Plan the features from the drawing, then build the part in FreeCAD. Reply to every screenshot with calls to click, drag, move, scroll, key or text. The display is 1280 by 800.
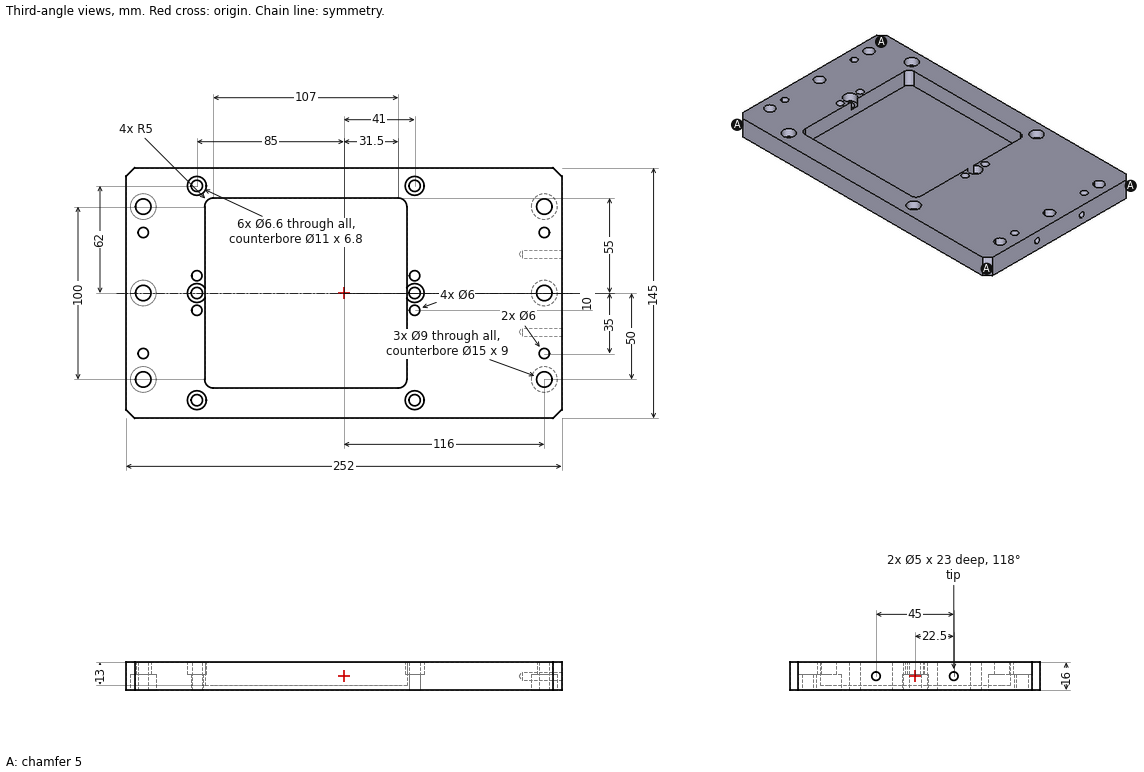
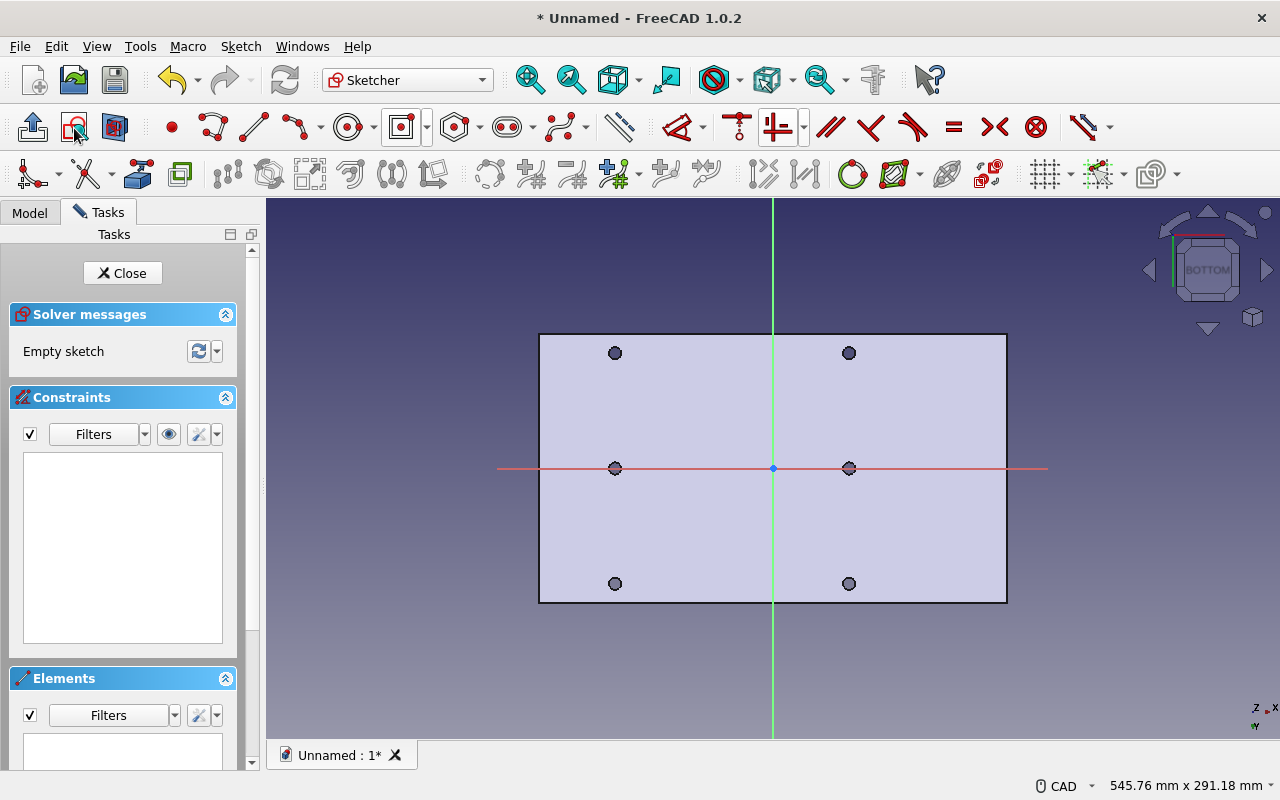
scroll(1104, 468, up, 3)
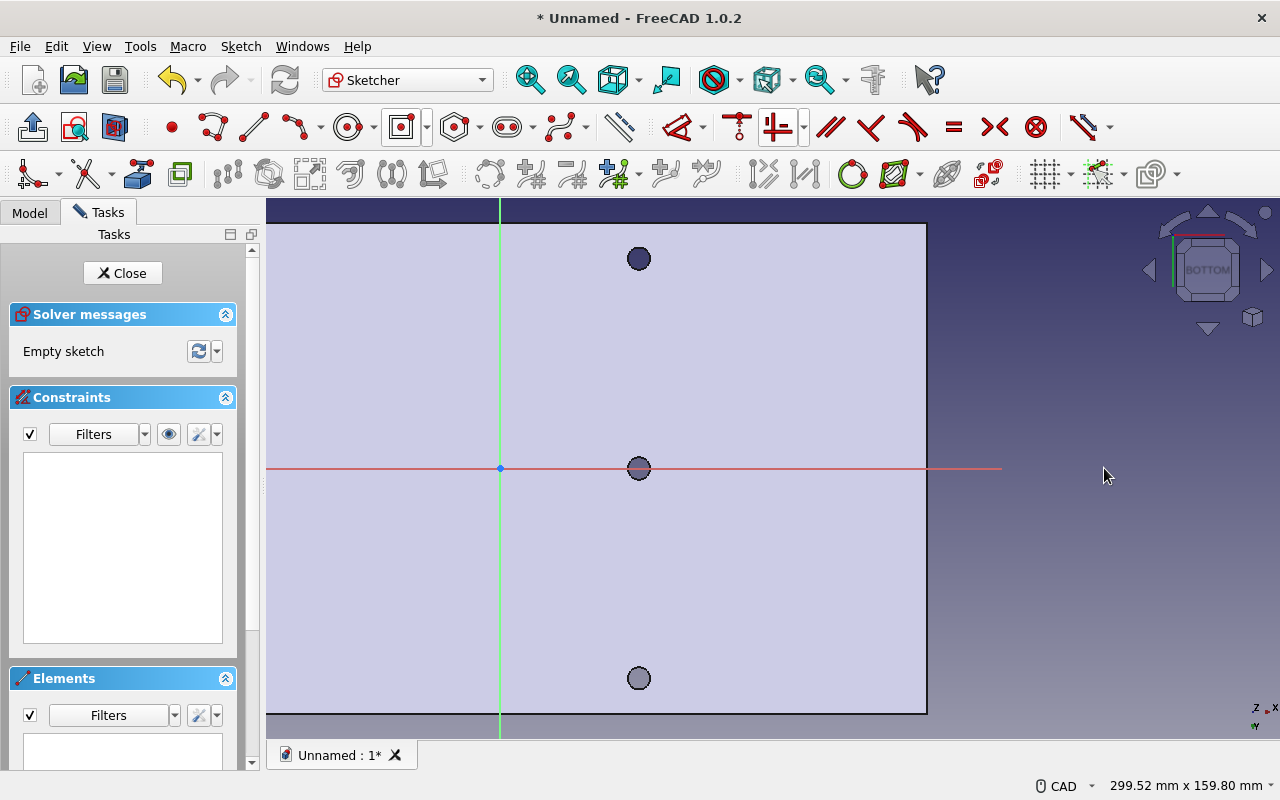
key(g)
key(c)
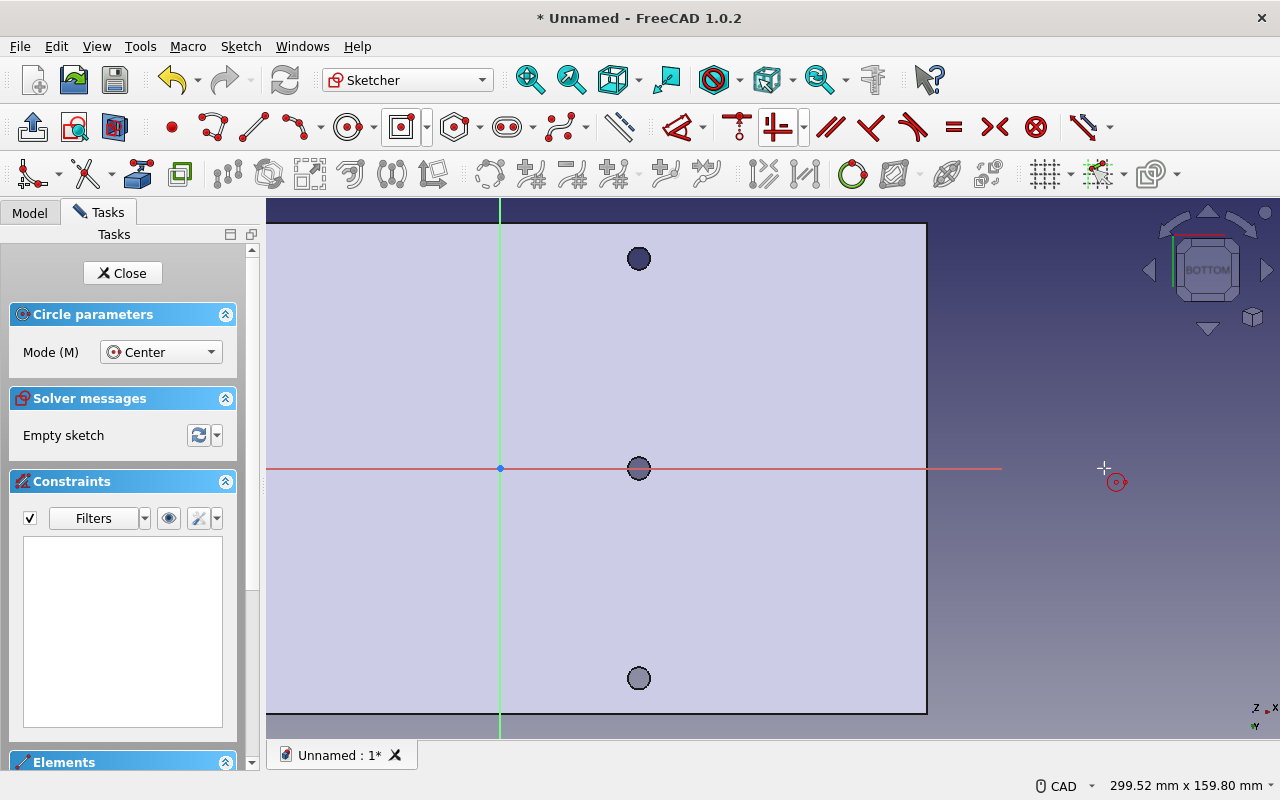
scroll(893, 299, up, 2)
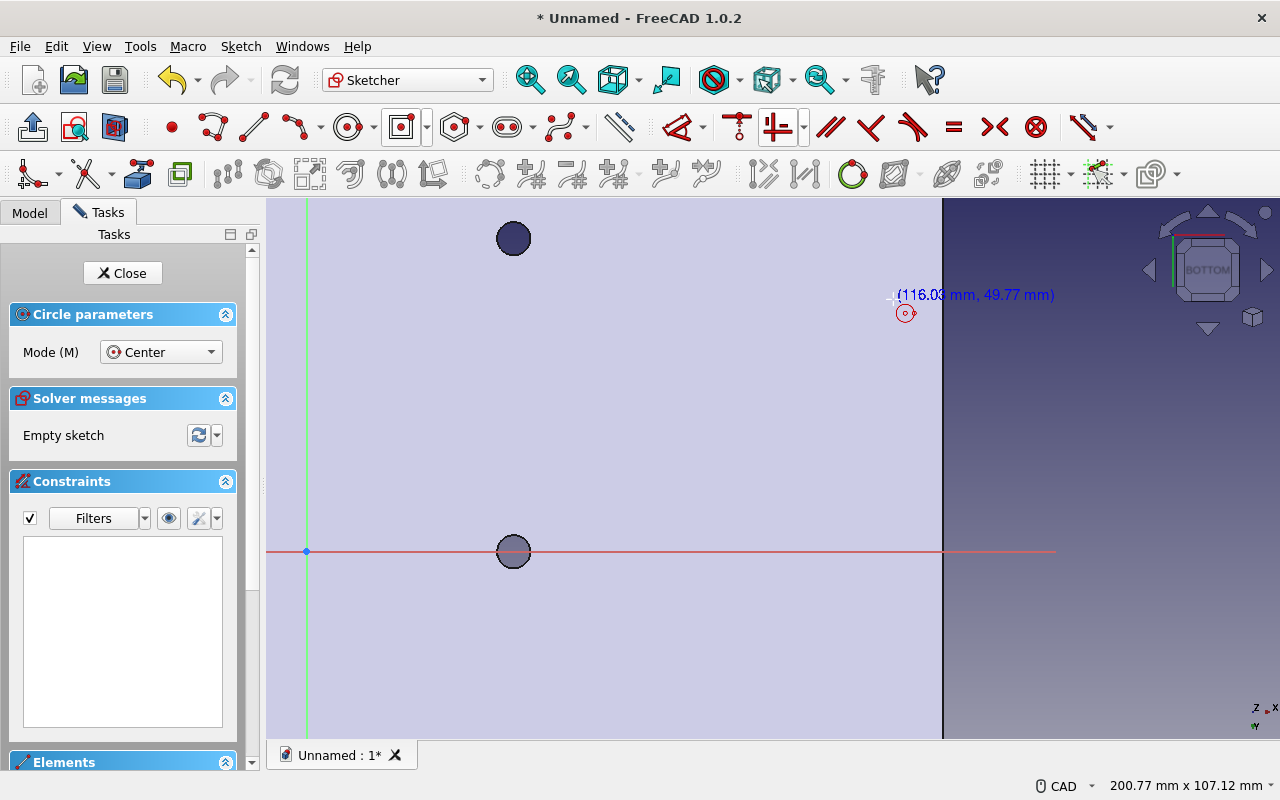
click(893, 299)
move(909, 283)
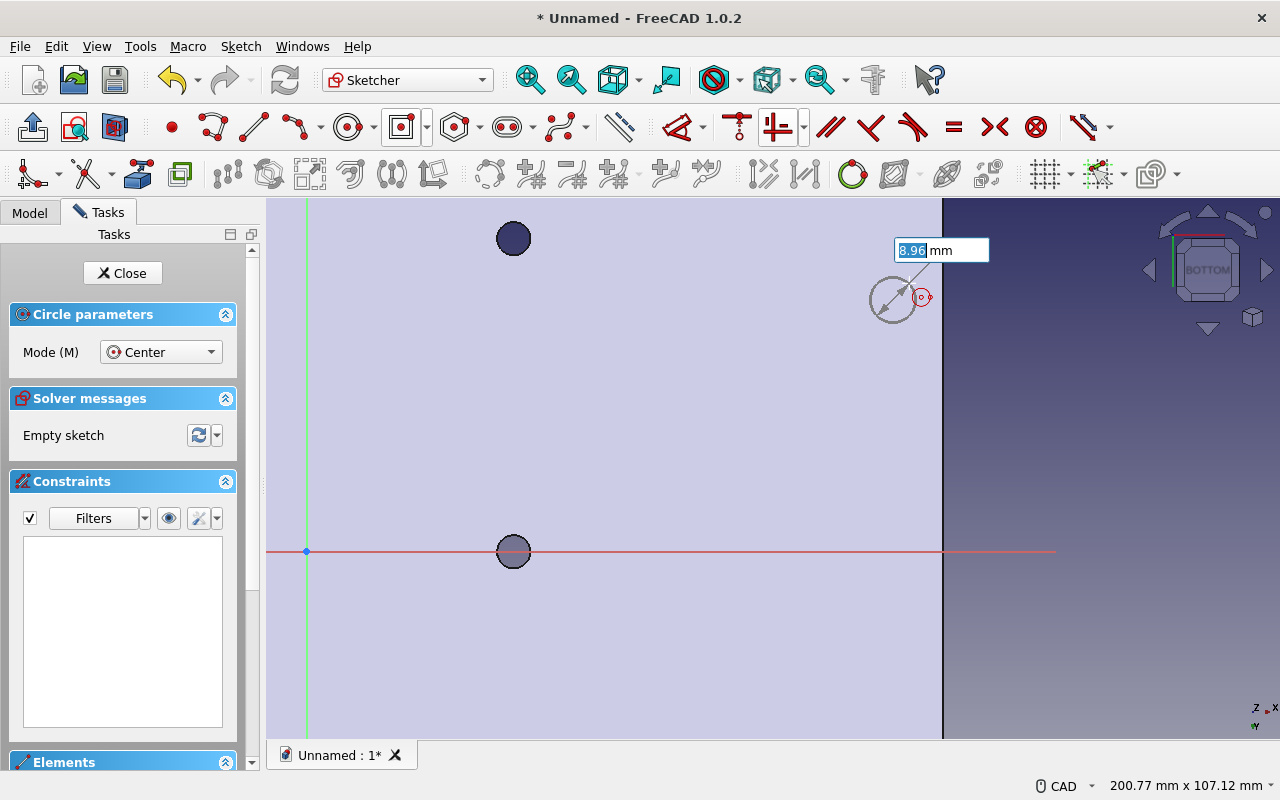
text(9)
key(Return)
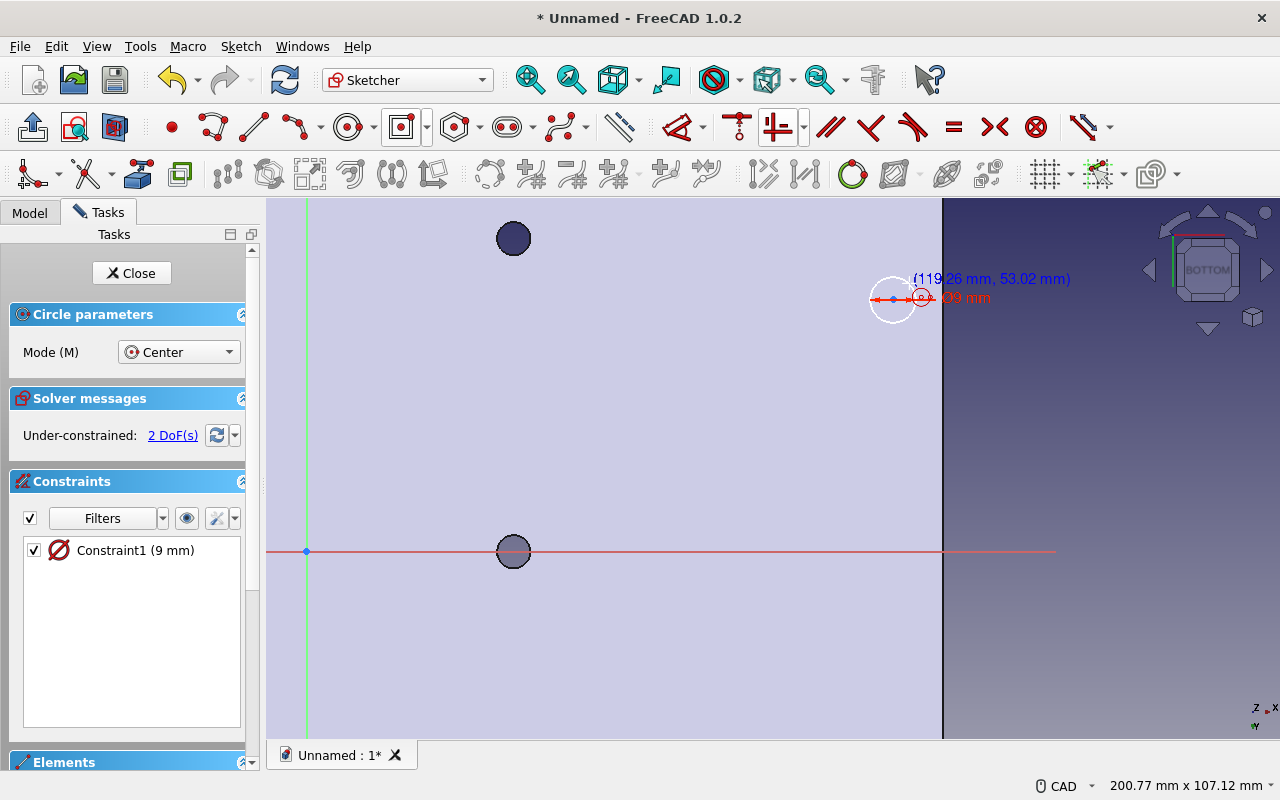
click(893, 552)
move(909, 536)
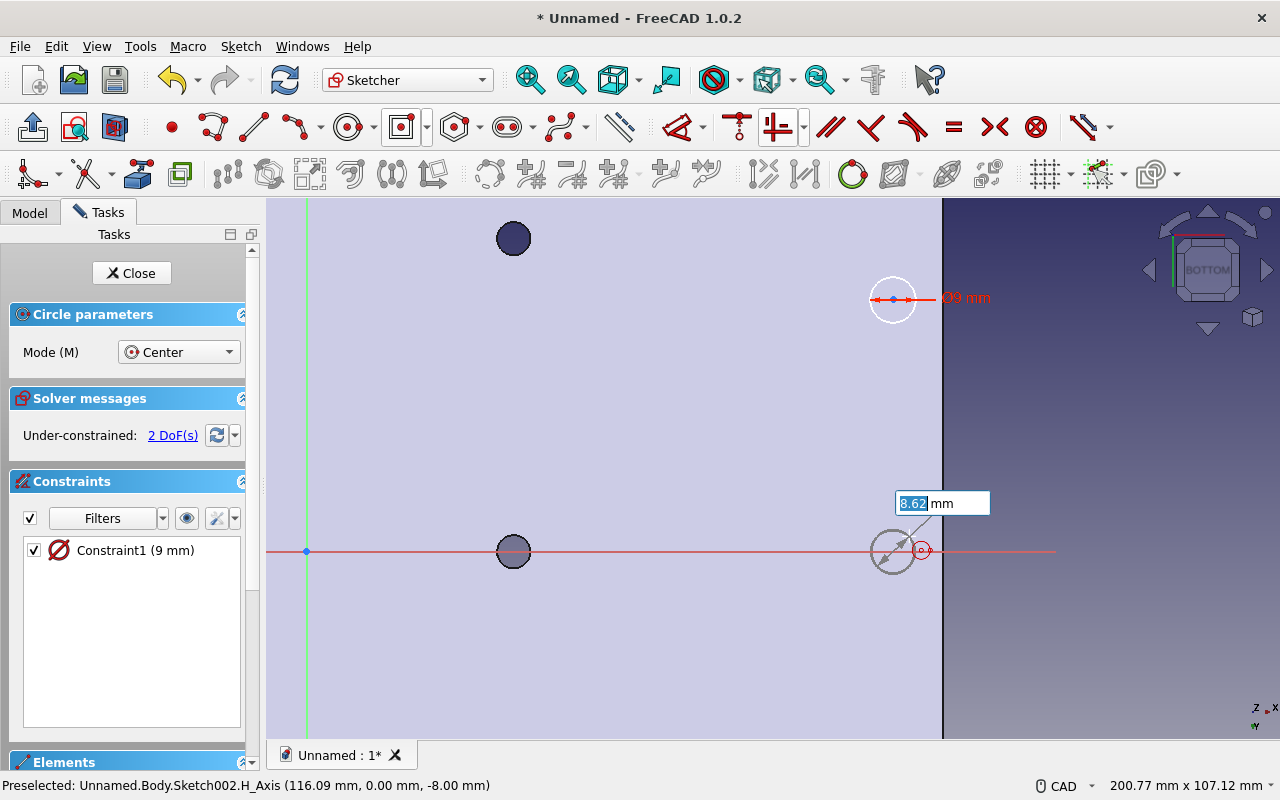
text(9)
key(Return)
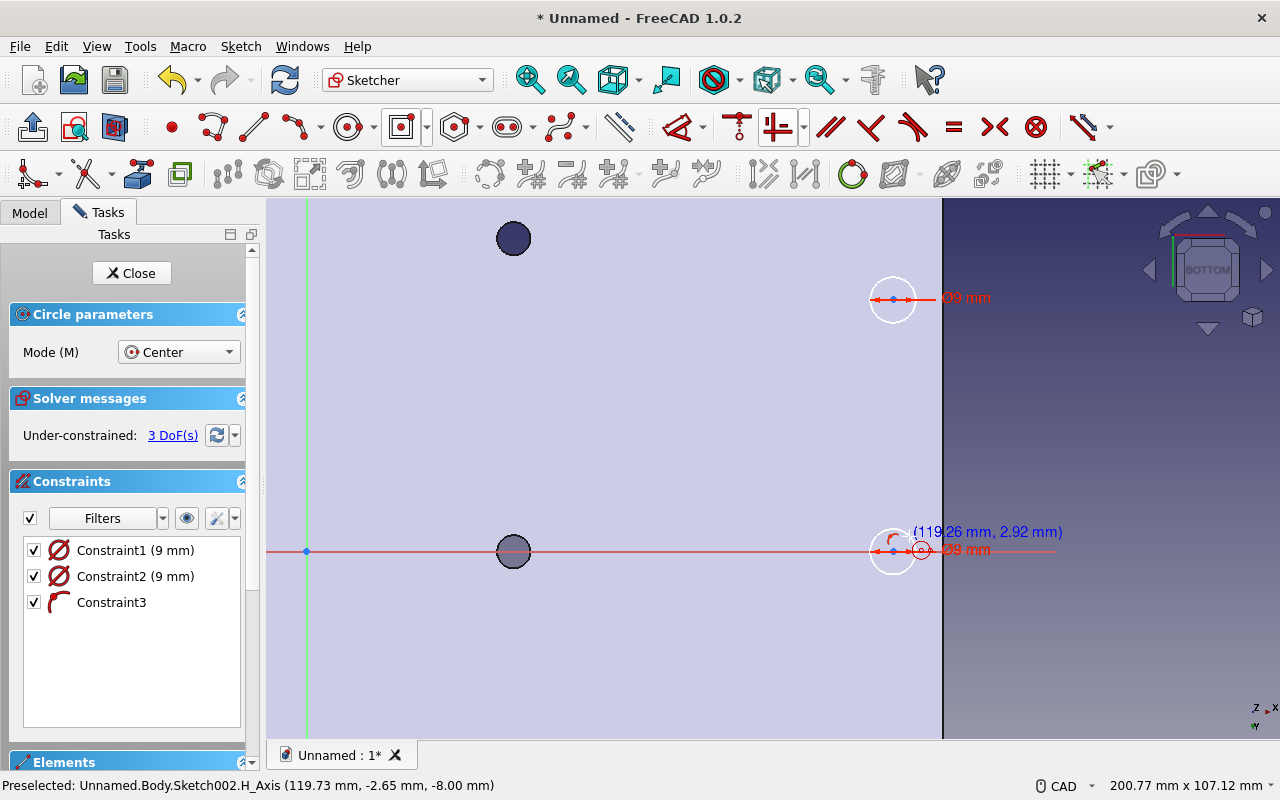
scroll(895, 299, down, 2)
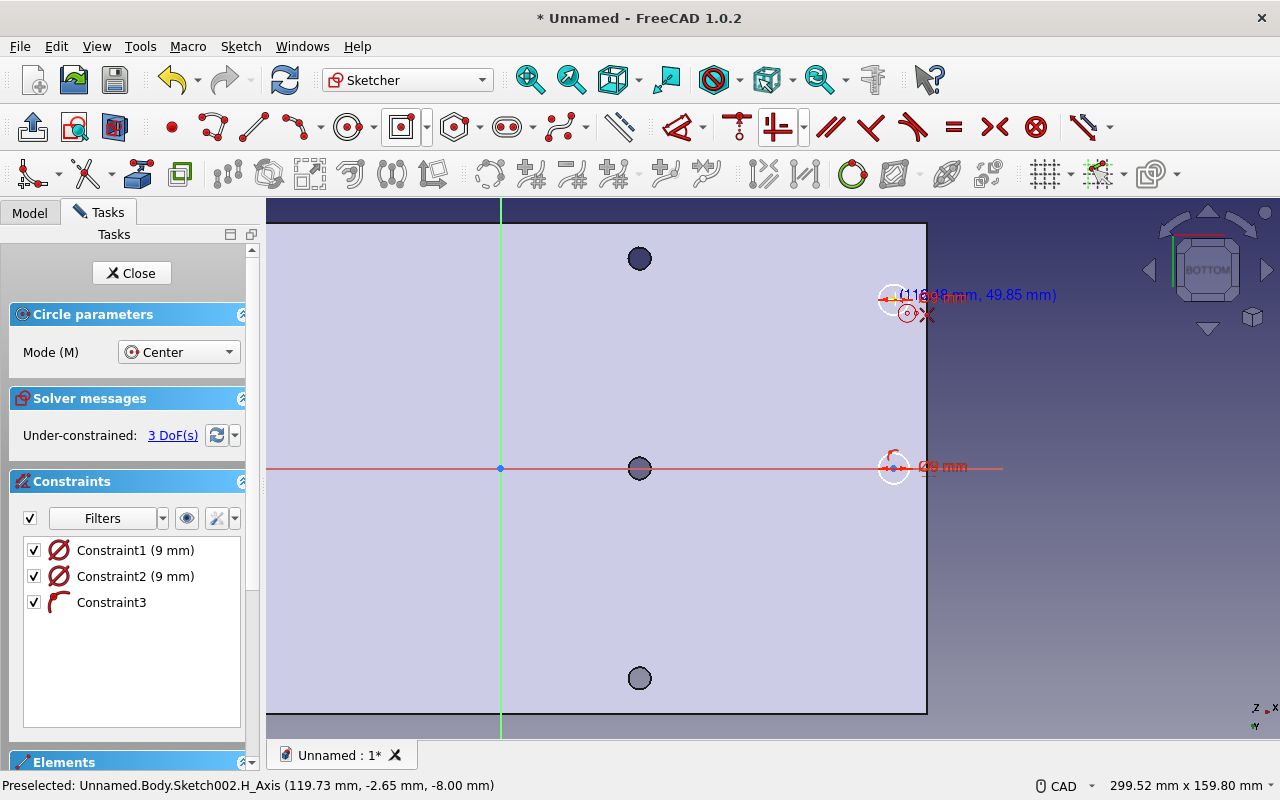
scroll(894, 638, up, 2)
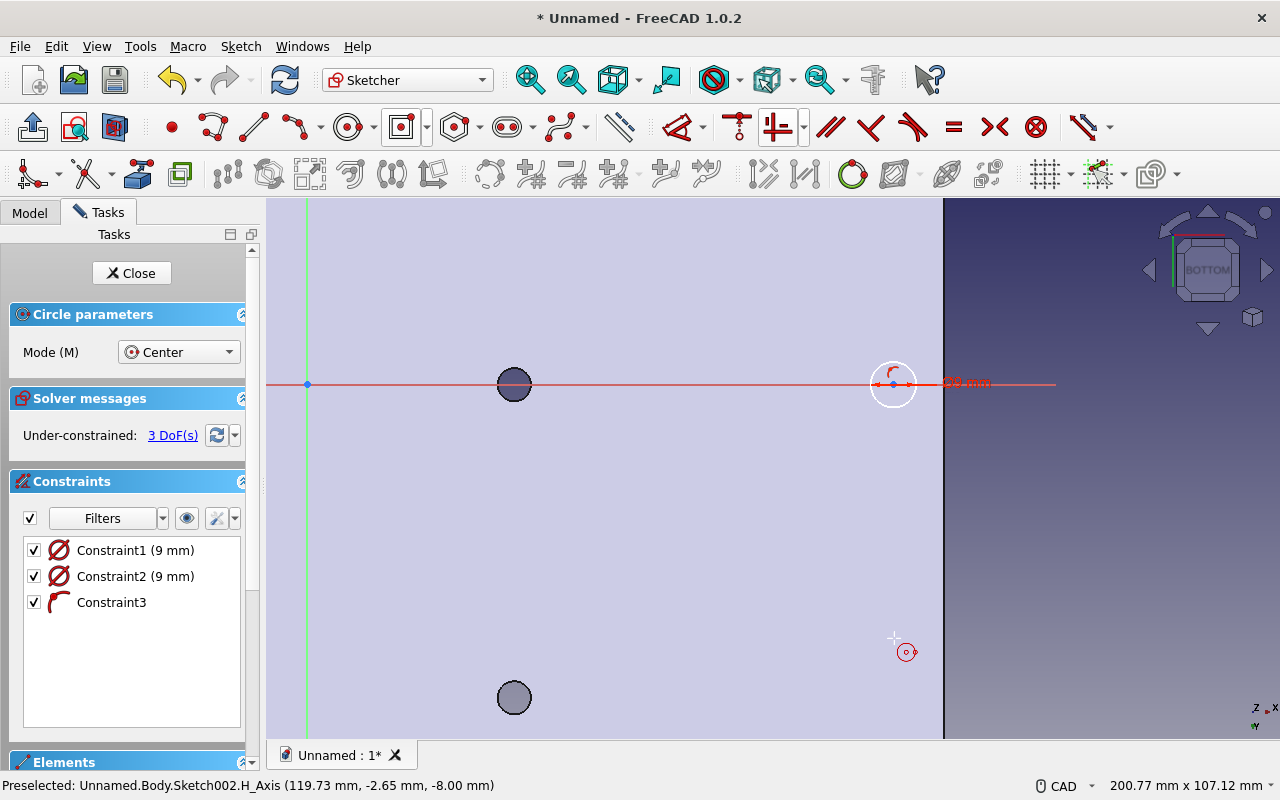
click(893, 637)
move(909, 621)